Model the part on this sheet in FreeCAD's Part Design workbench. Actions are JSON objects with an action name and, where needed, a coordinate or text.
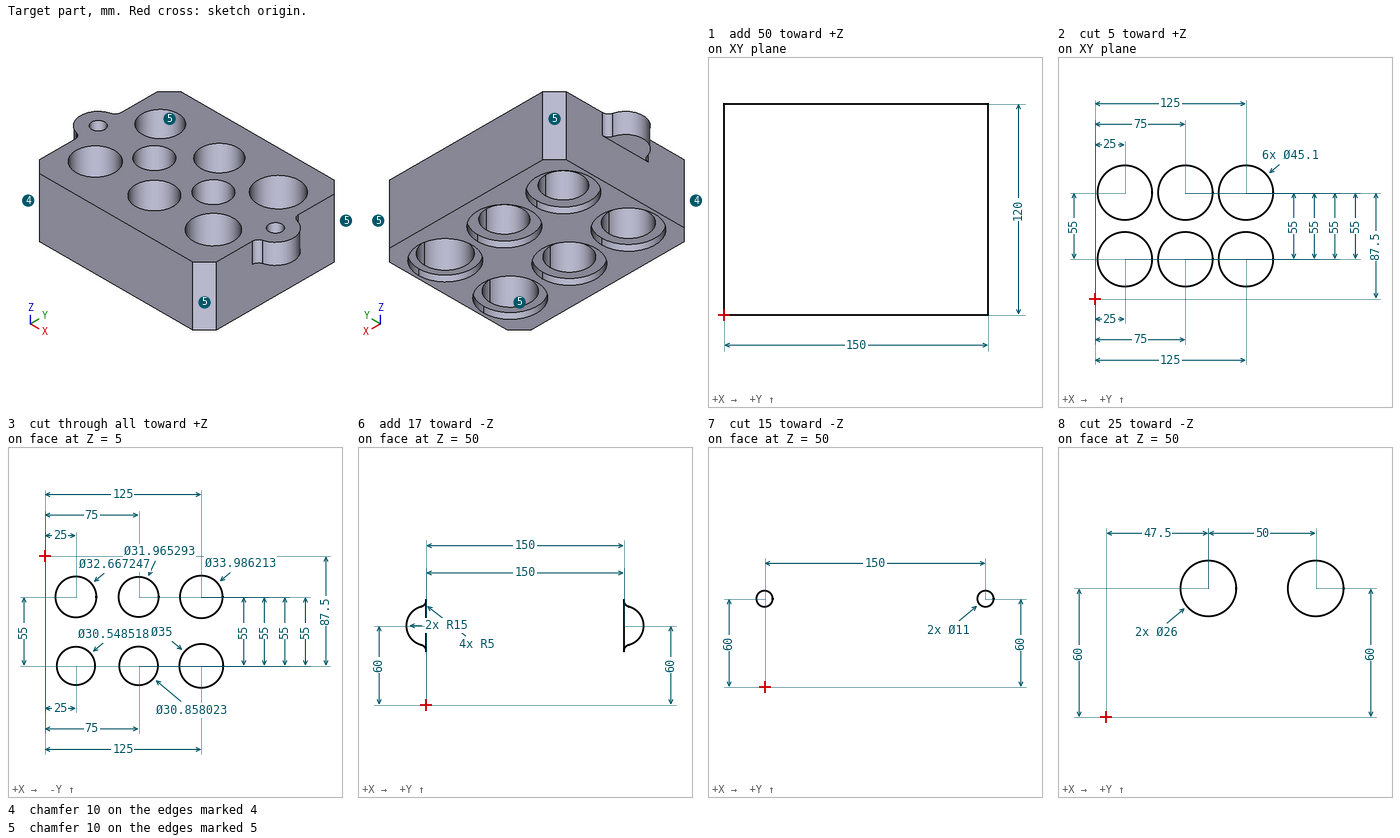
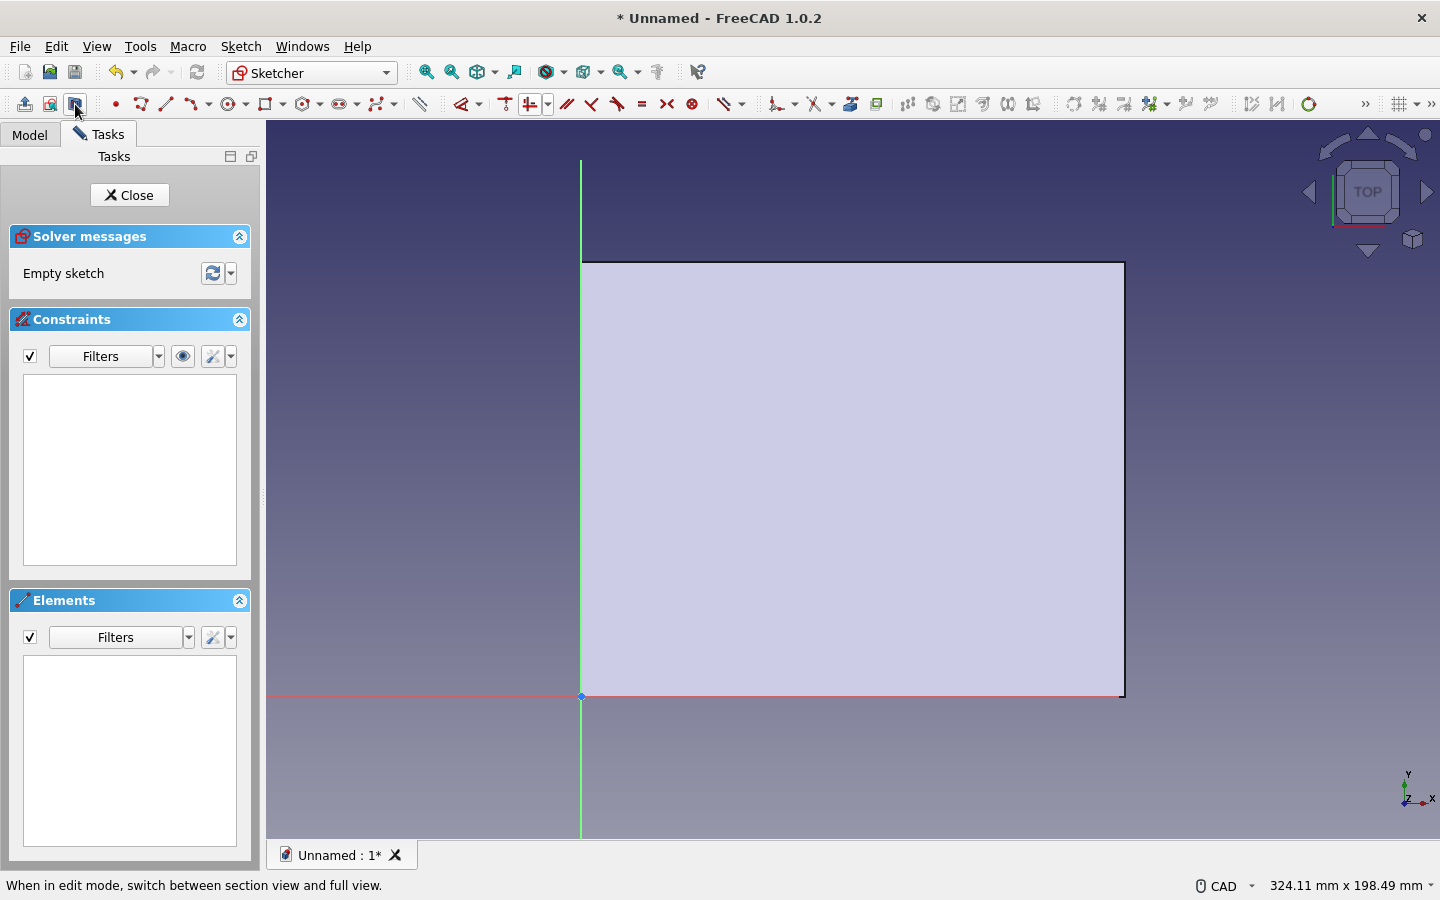
{"action": "key", "text": "g c"}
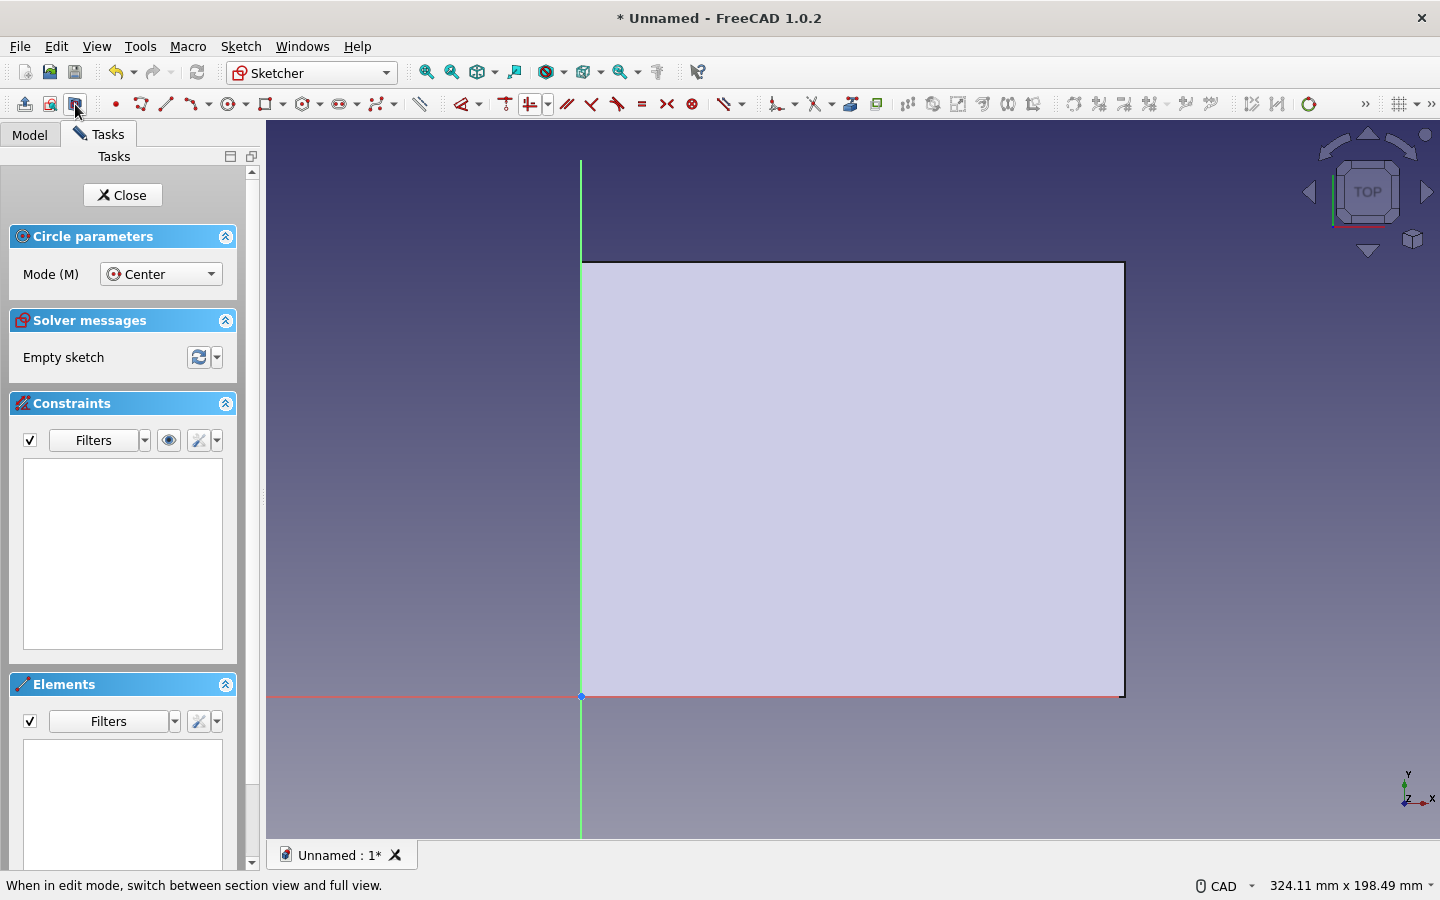
{"action": "left_click", "coordinate": [1034, 380]}
{"action": "left_click", "coordinate": [1092, 322]}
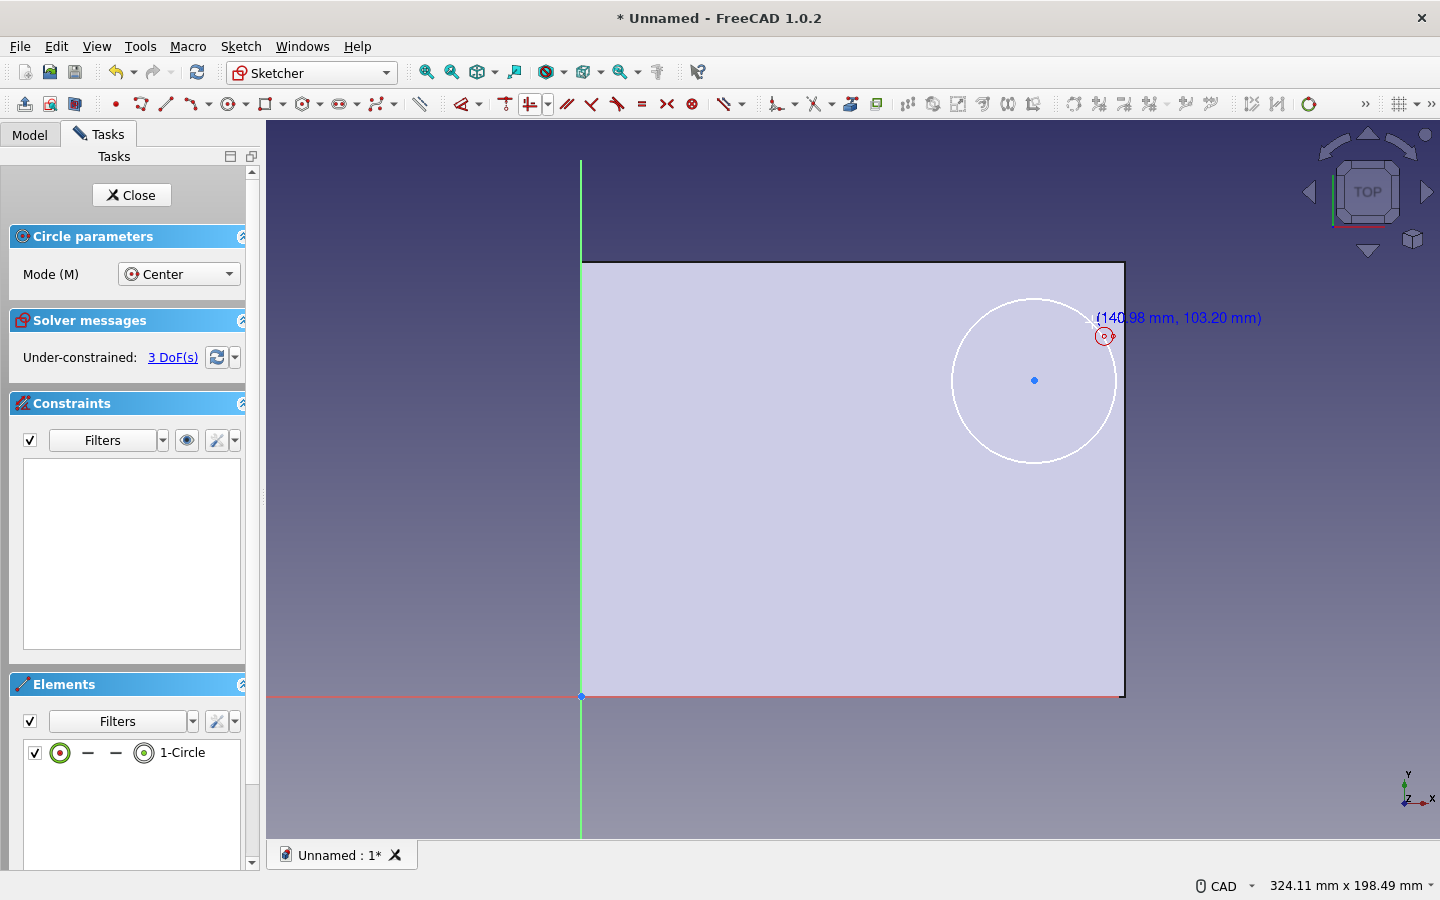
{"action": "left_click", "coordinate": [853, 380]}
{"action": "left_click", "coordinate": [911, 322]}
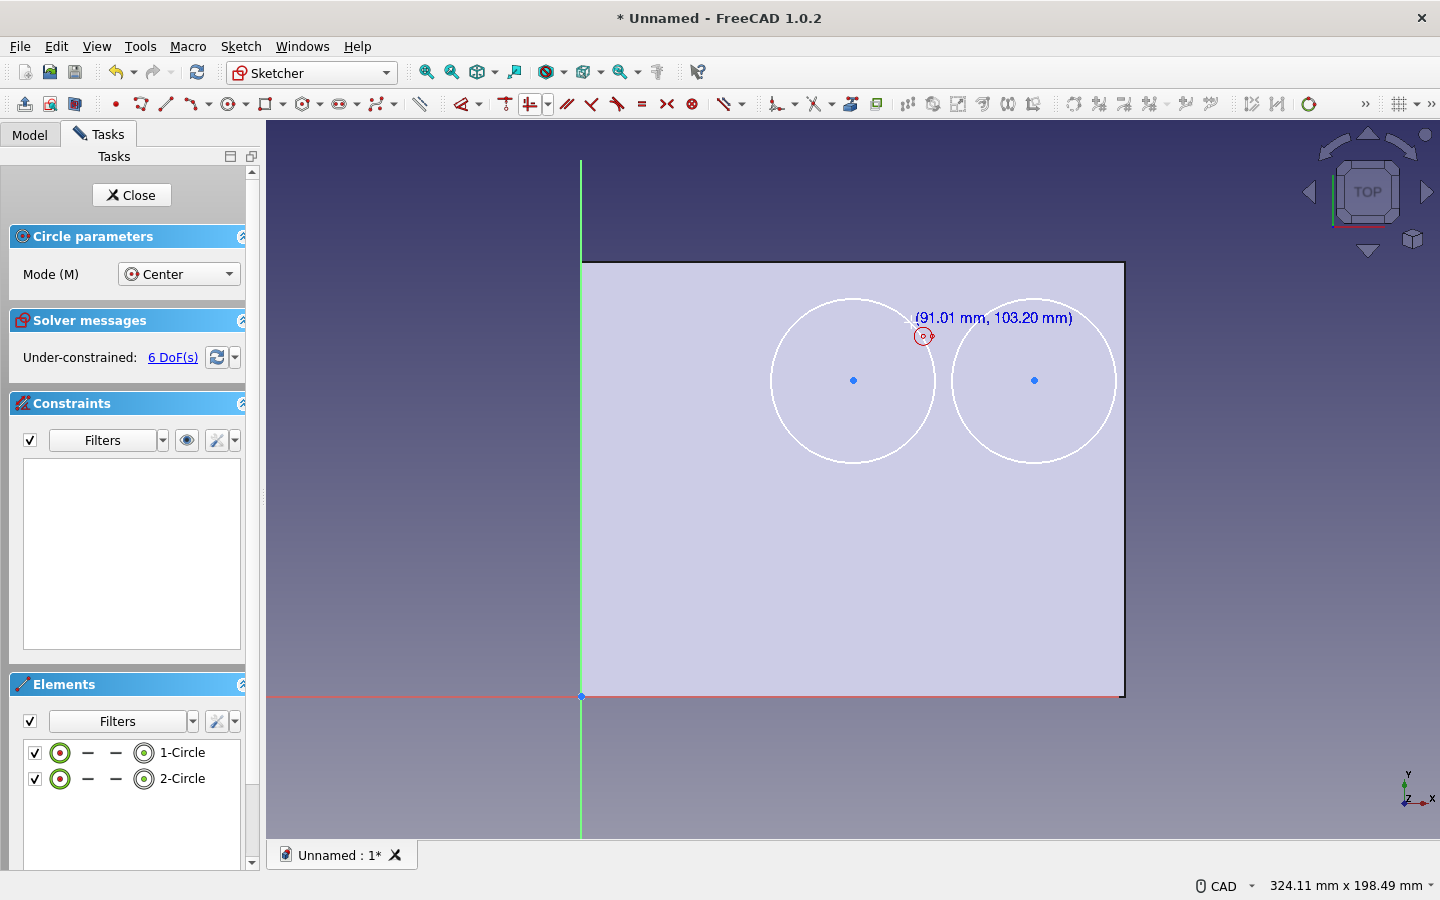
{"action": "left_click", "coordinate": [672, 380]}
{"action": "left_click", "coordinate": [730, 322]}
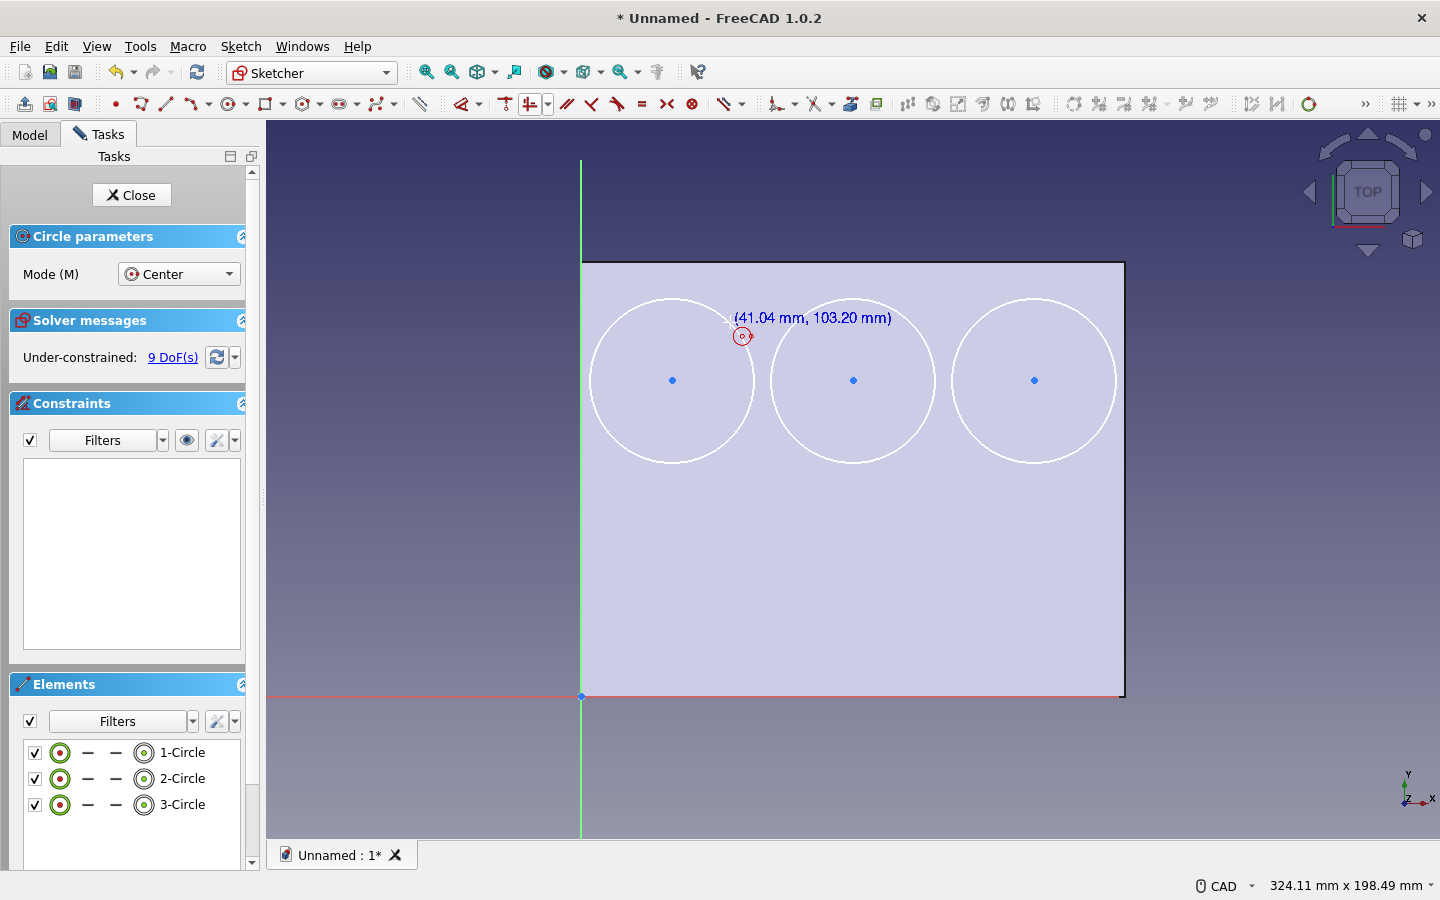
{"action": "left_click", "coordinate": [672, 579]}
{"action": "left_click", "coordinate": [730, 521]}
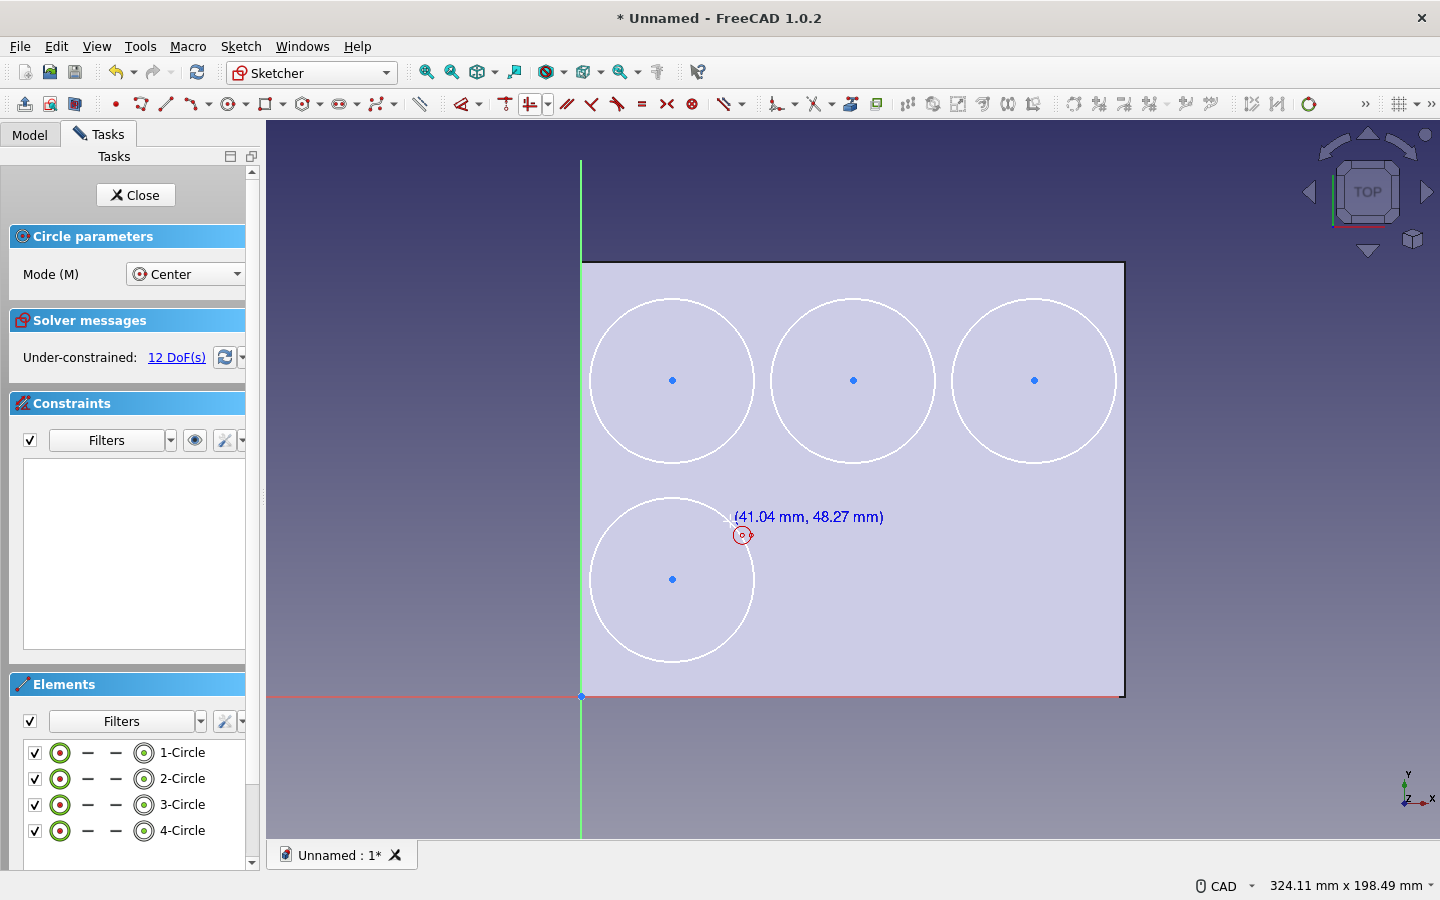
{"action": "left_click", "coordinate": [853, 579]}
{"action": "left_click", "coordinate": [911, 521]}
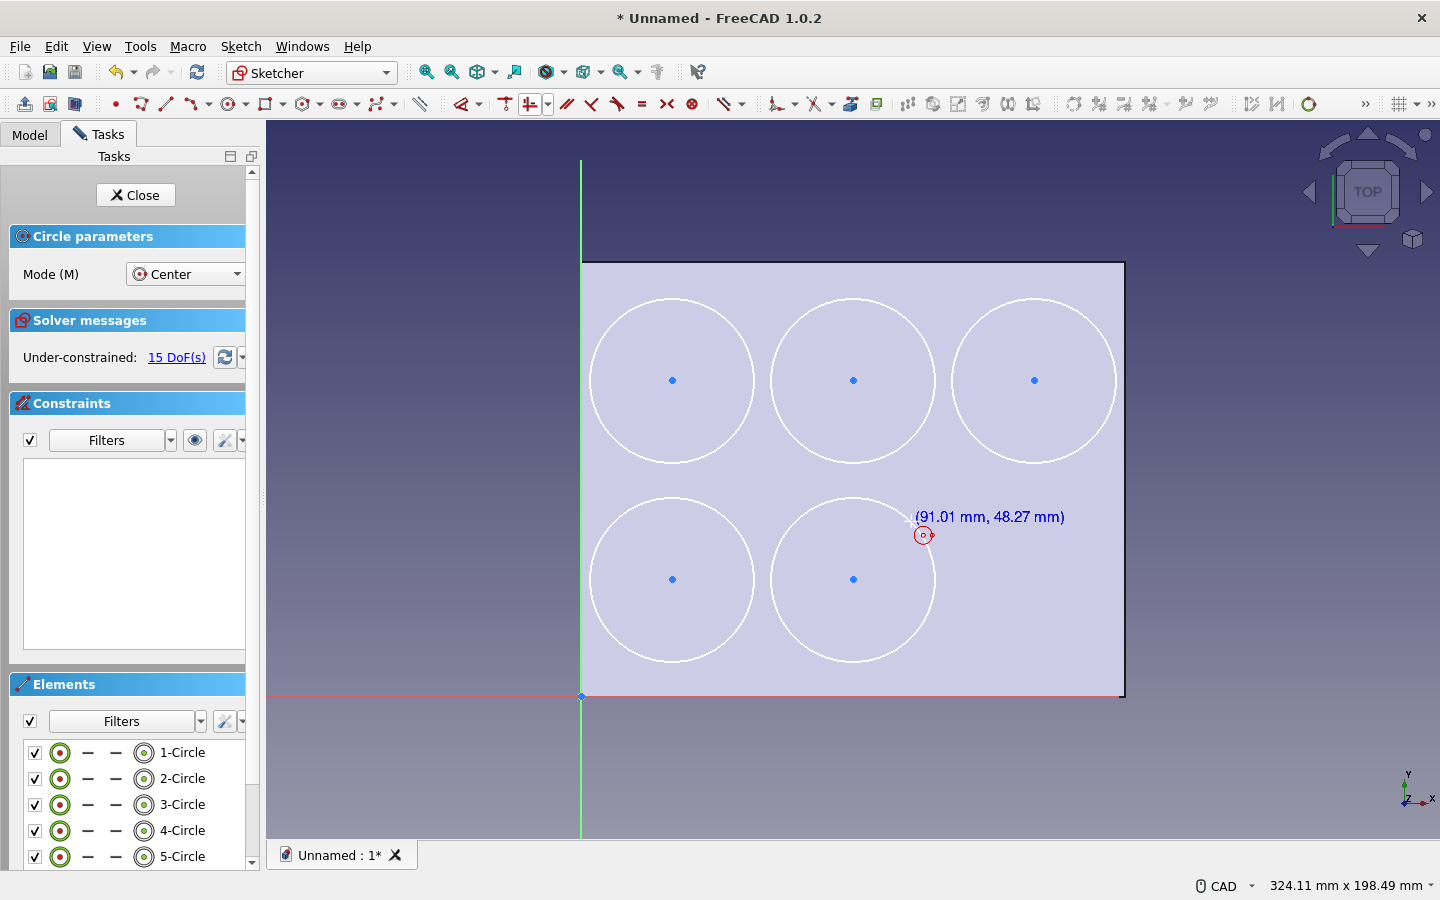
{"action": "left_click", "coordinate": [1034, 579]}
{"action": "left_click", "coordinate": [1092, 521]}
{"action": "key", "text": "Escape"}